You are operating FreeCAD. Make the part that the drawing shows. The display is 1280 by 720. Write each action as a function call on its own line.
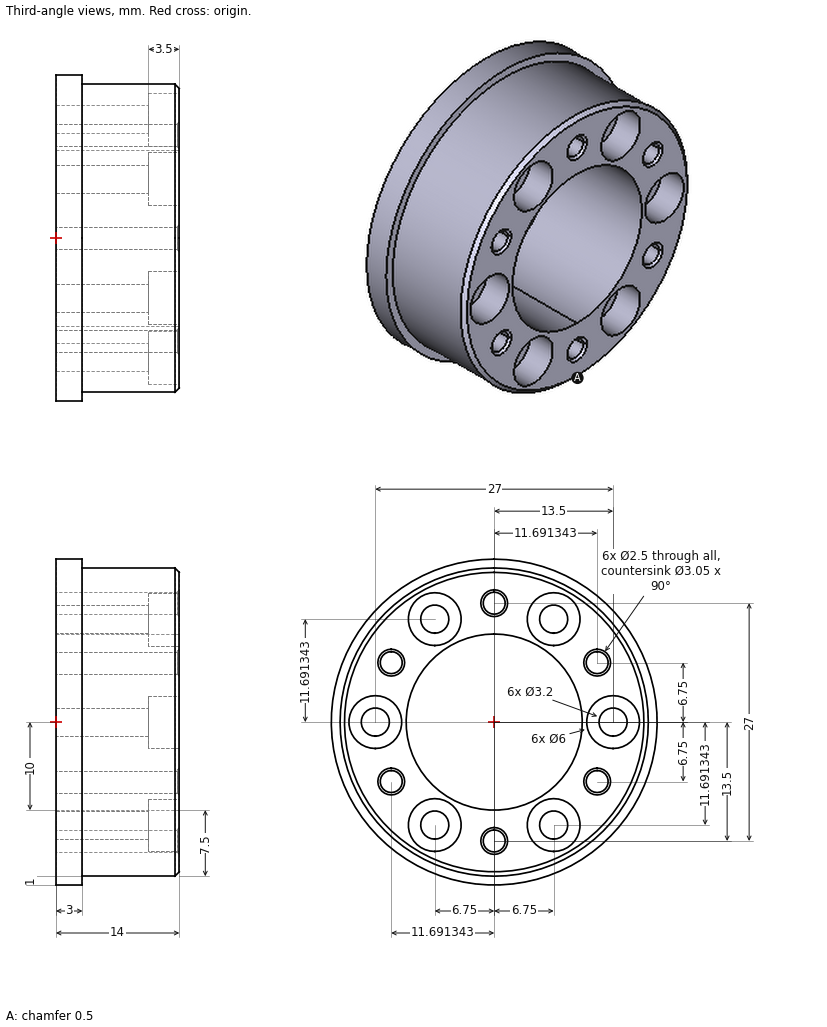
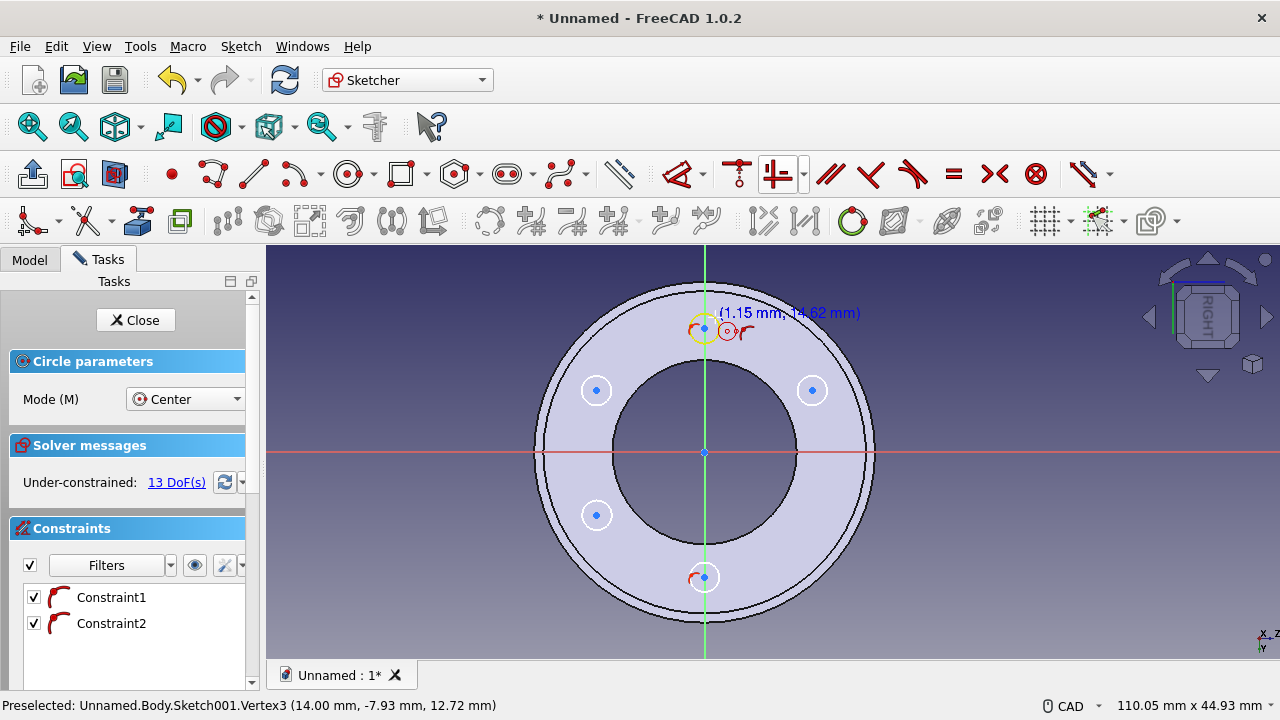
scroll(812, 514, up, 3)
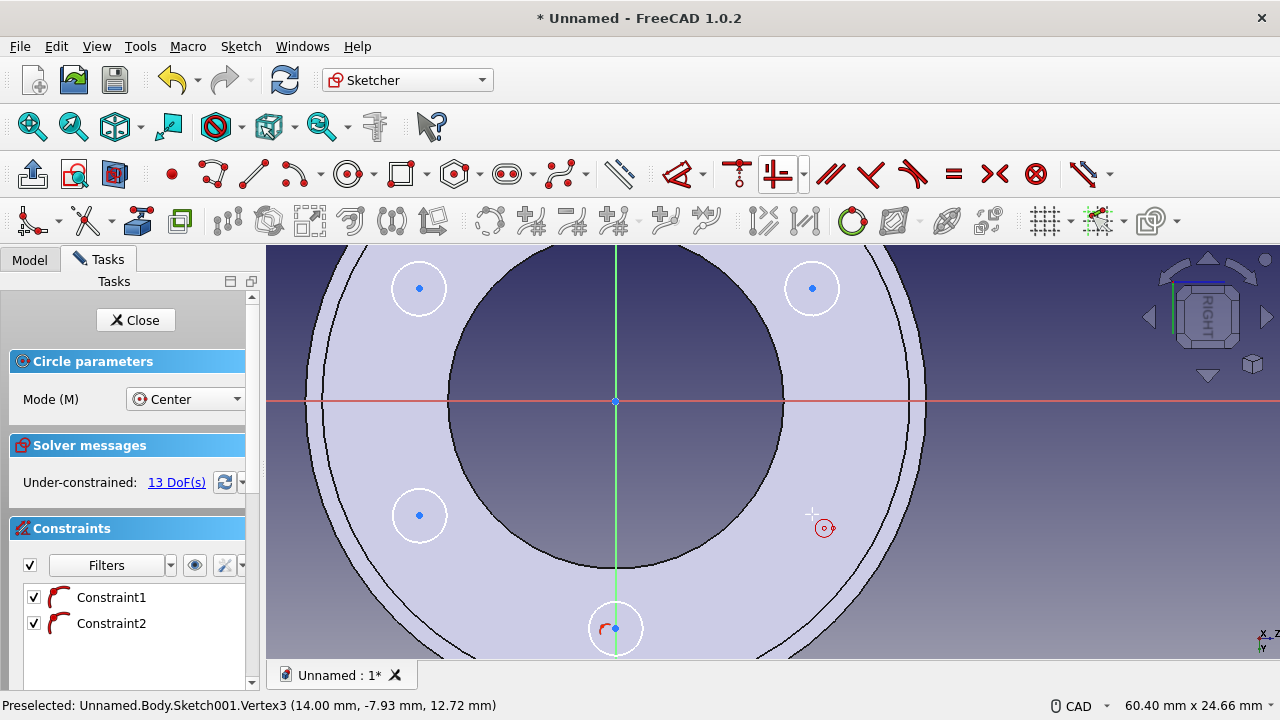
click(812, 514)
click(831, 495)
key(Escape)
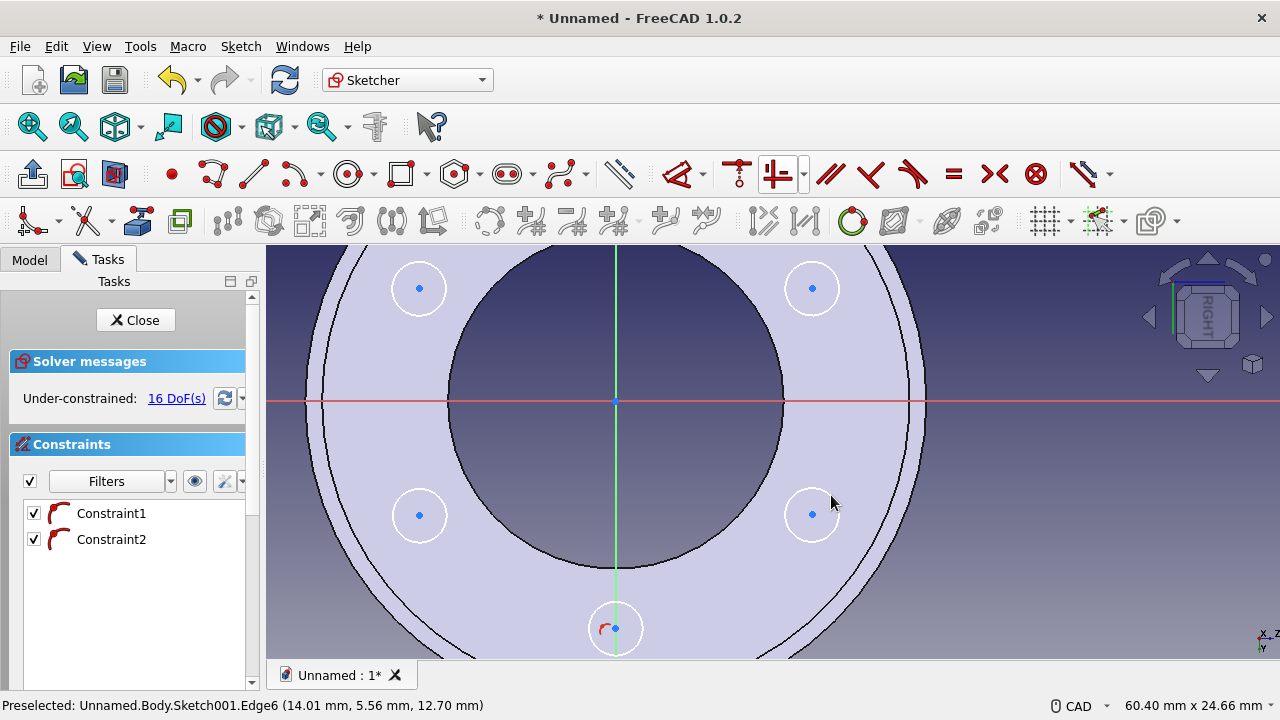
click(635, 610)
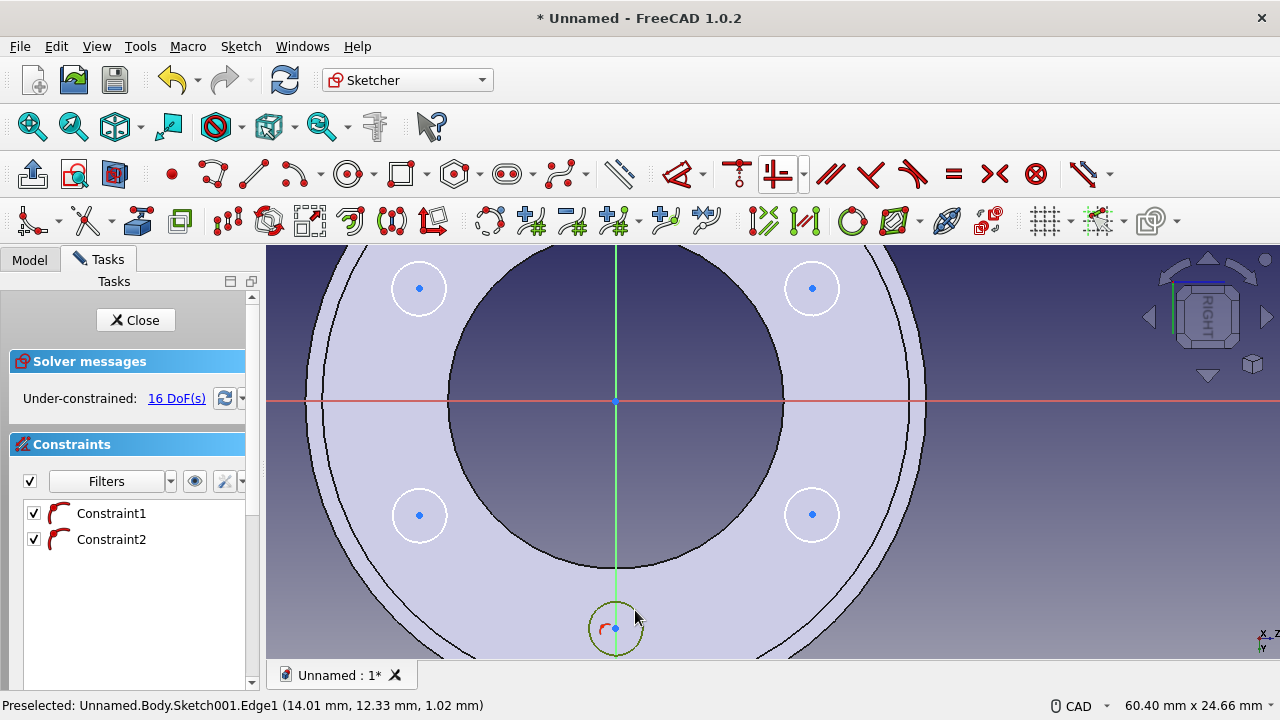
click(439, 497)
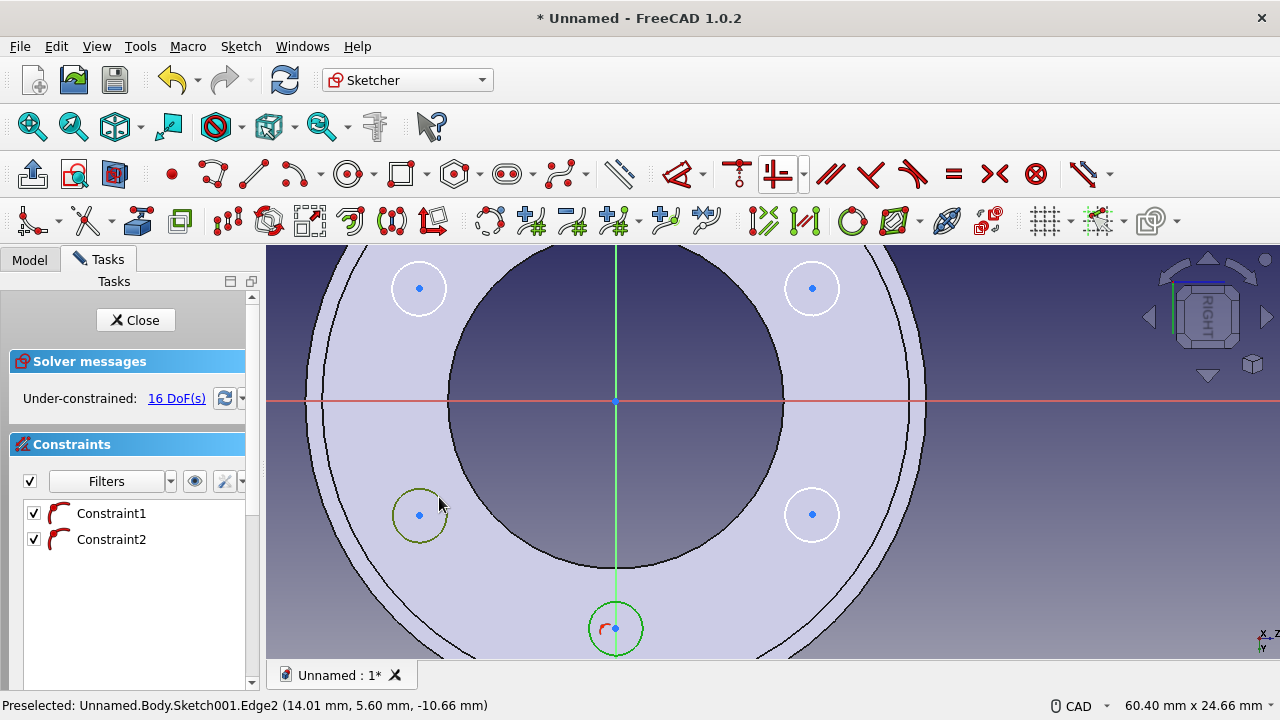
click(400, 308)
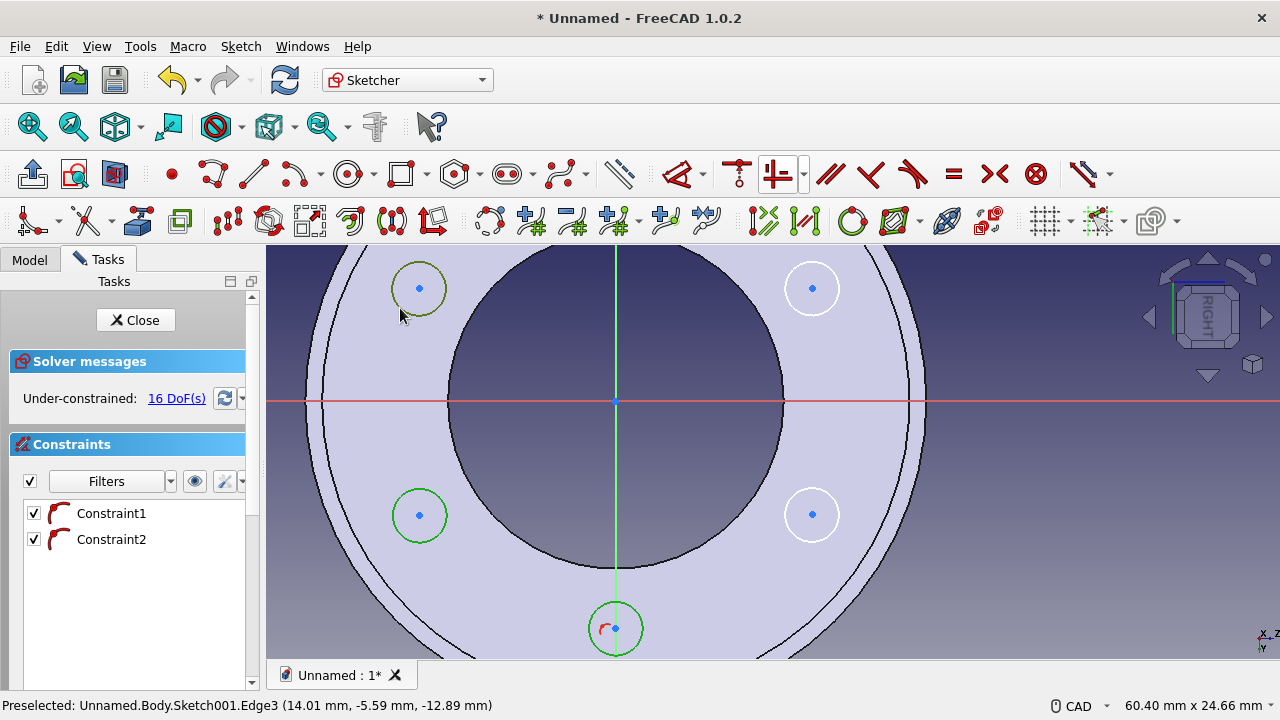
scroll(812, 514, down, 3)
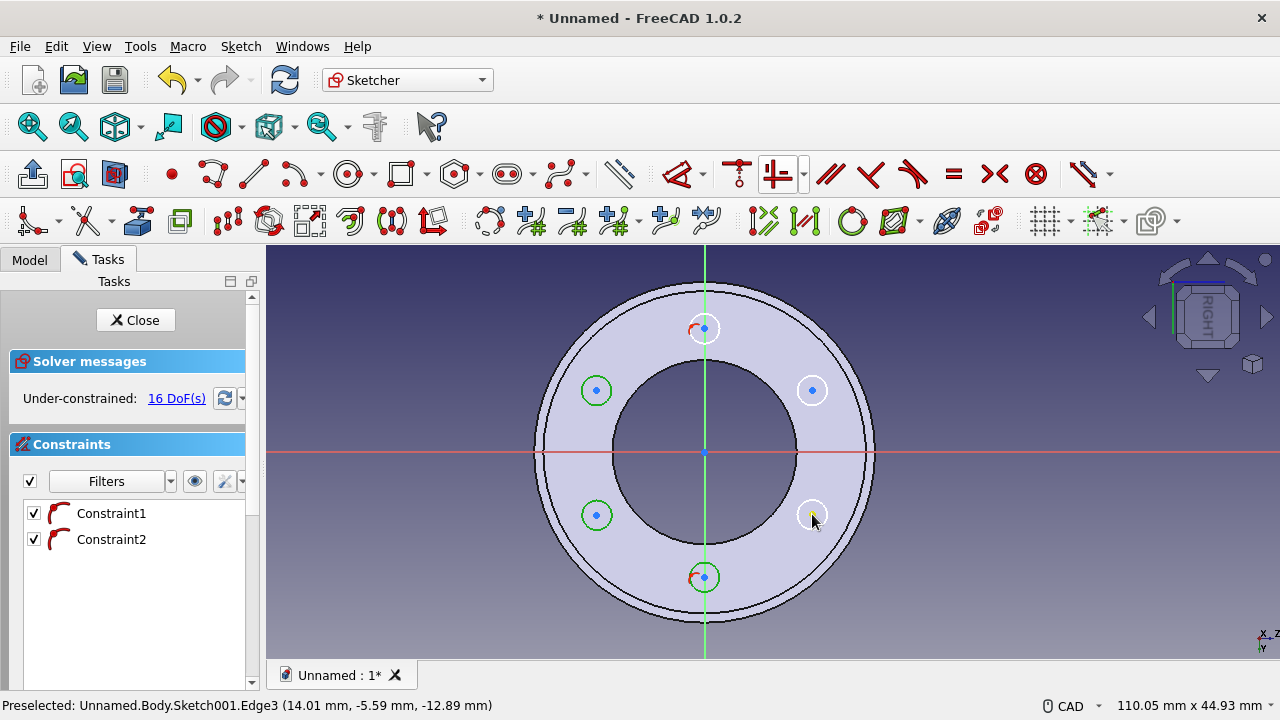
scroll(715, 318, up, 2)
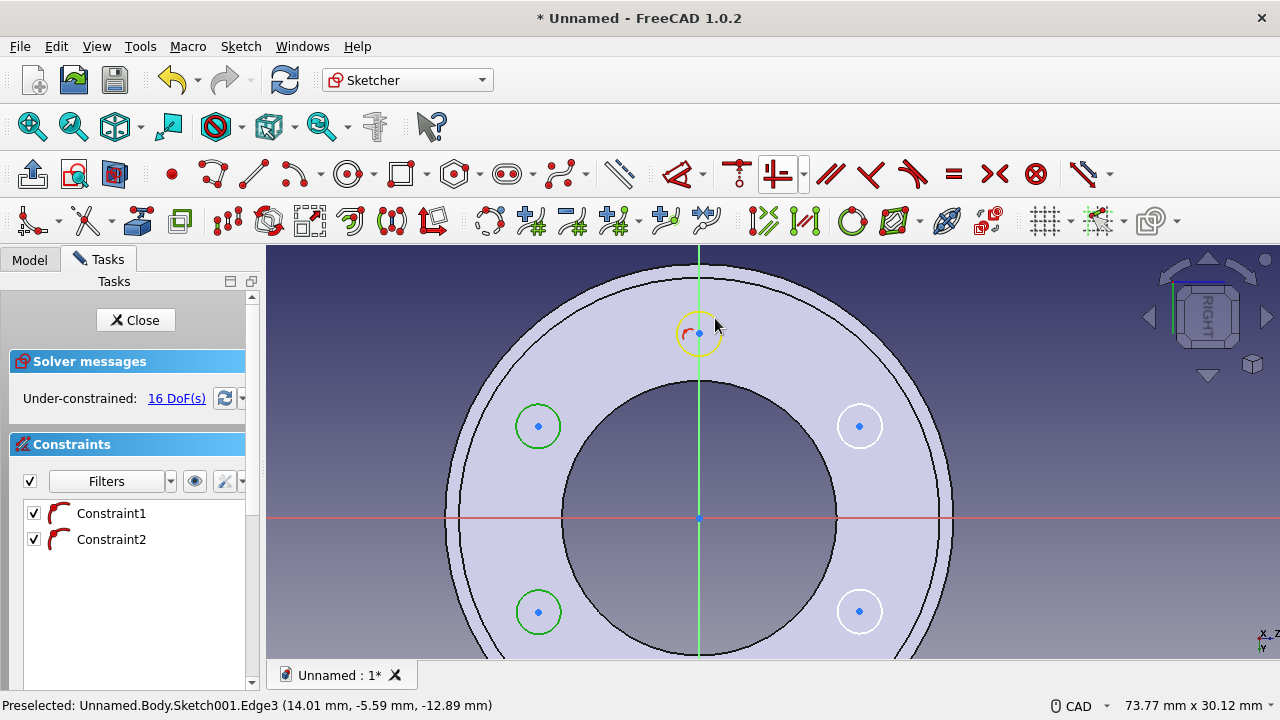
click(715, 318)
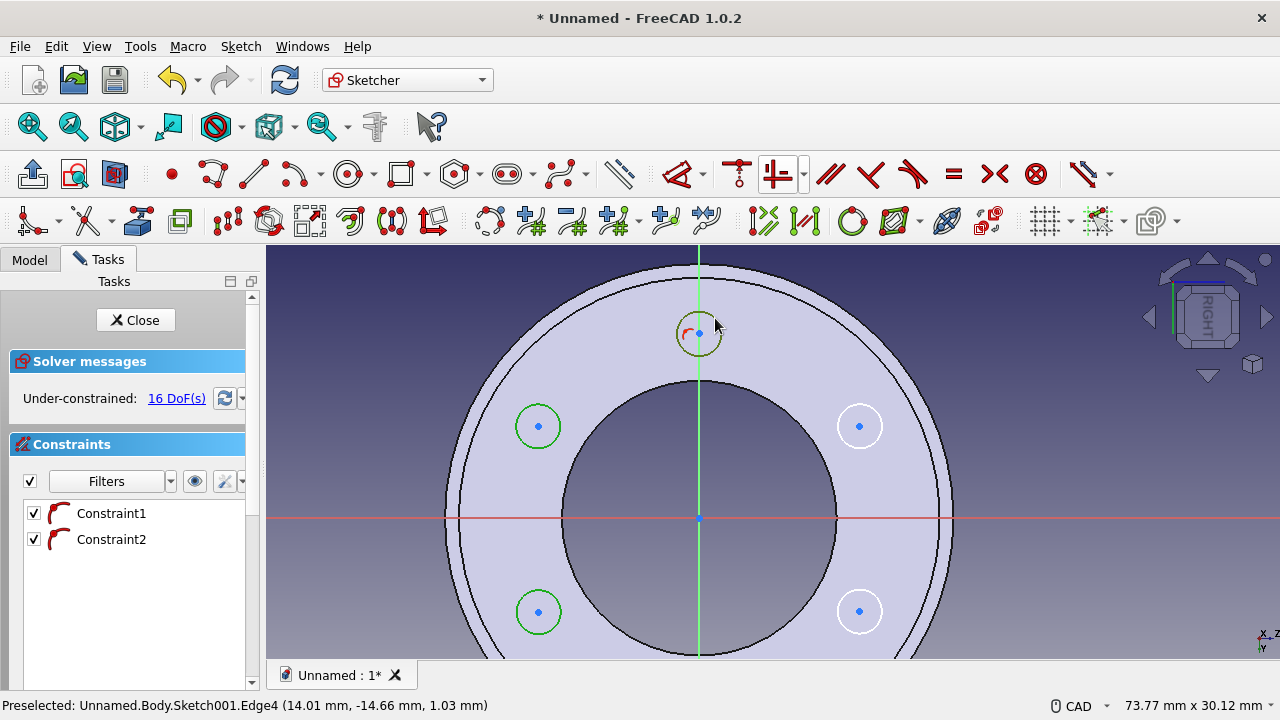
click(876, 411)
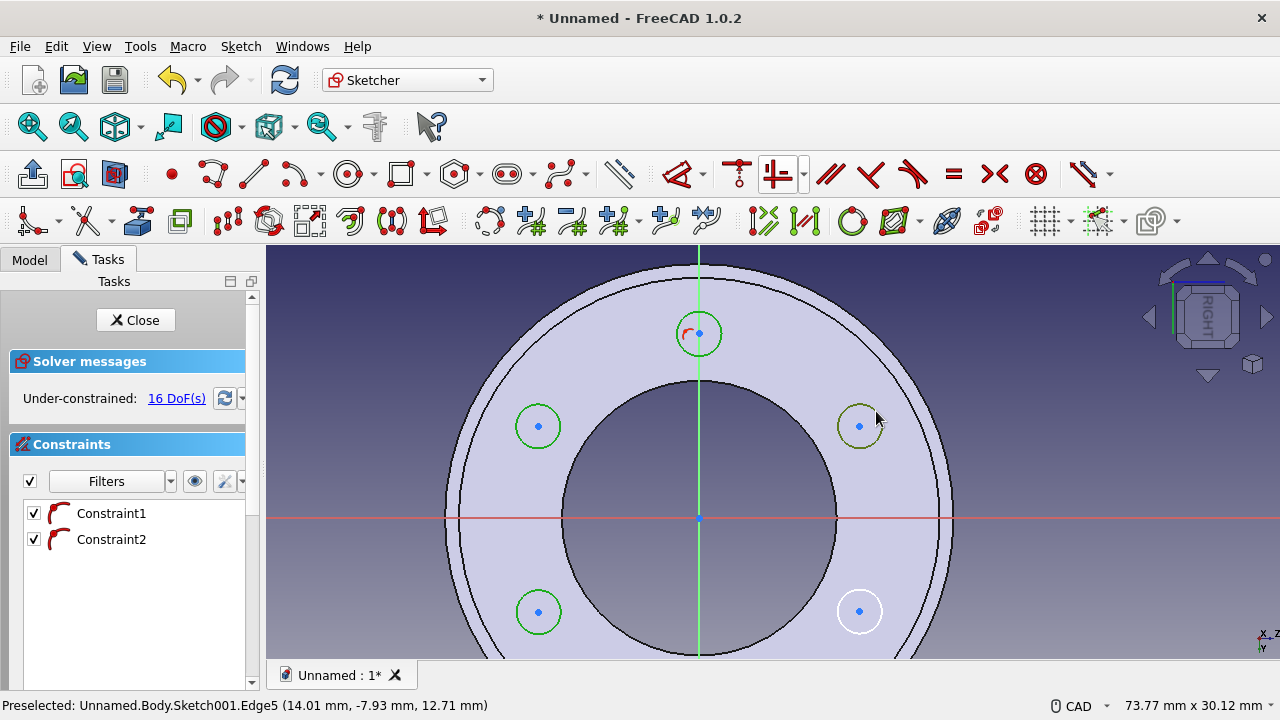
click(875, 596)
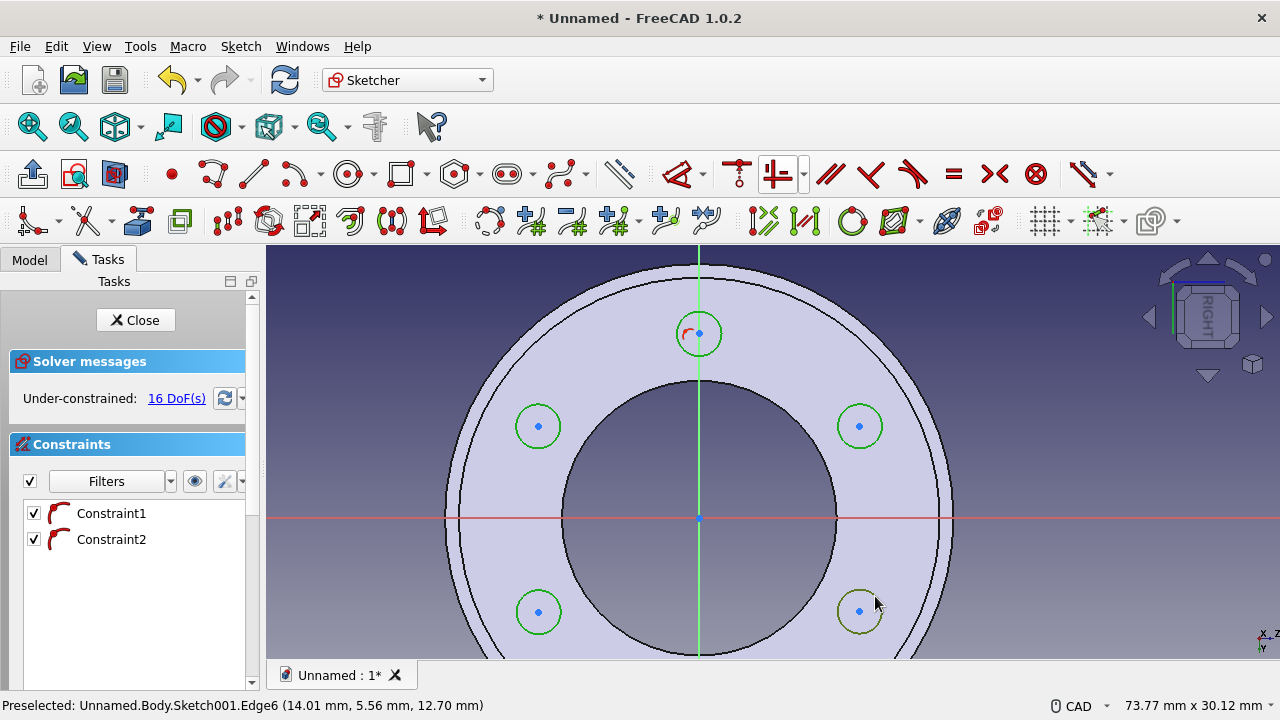
click(954, 174)